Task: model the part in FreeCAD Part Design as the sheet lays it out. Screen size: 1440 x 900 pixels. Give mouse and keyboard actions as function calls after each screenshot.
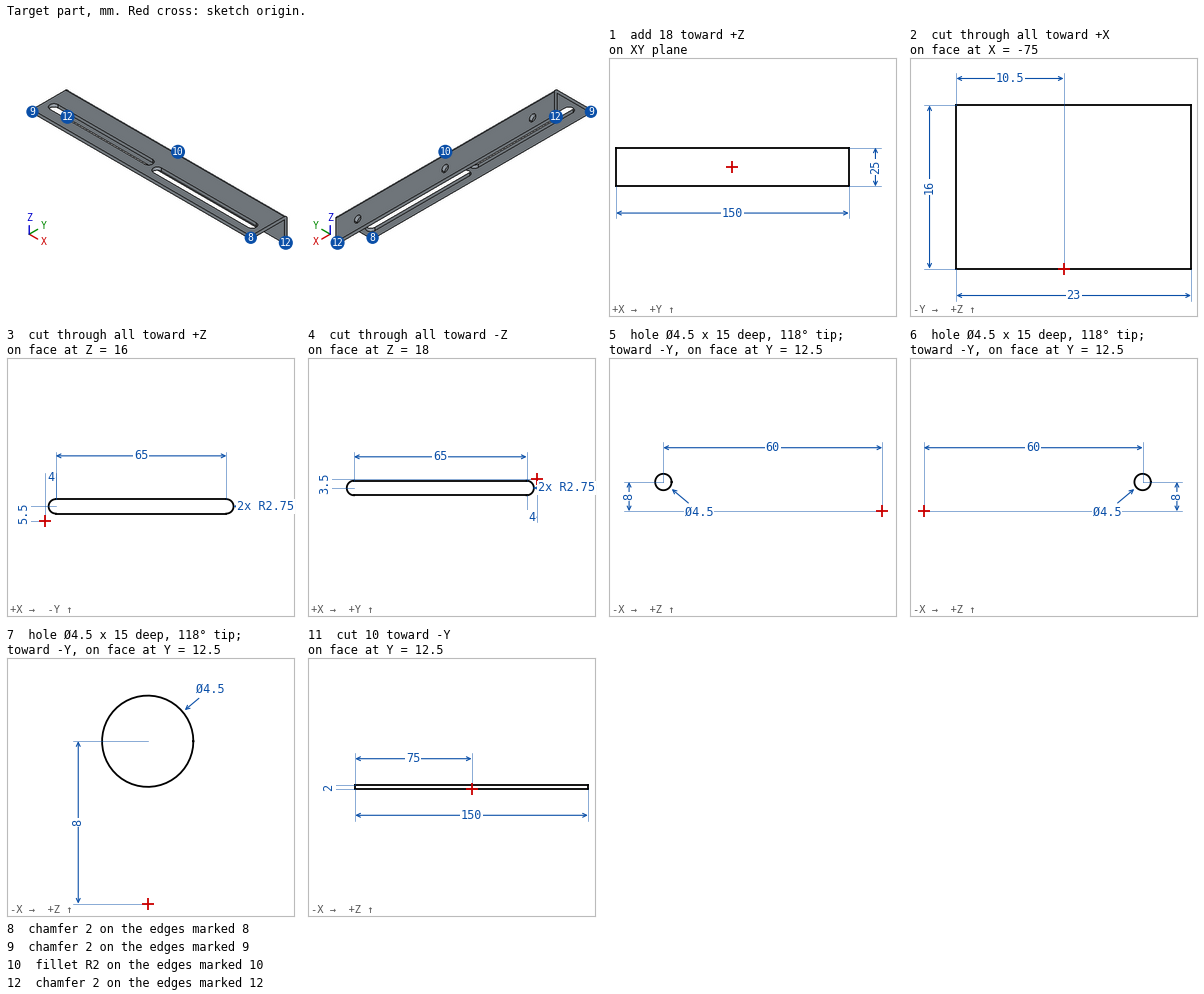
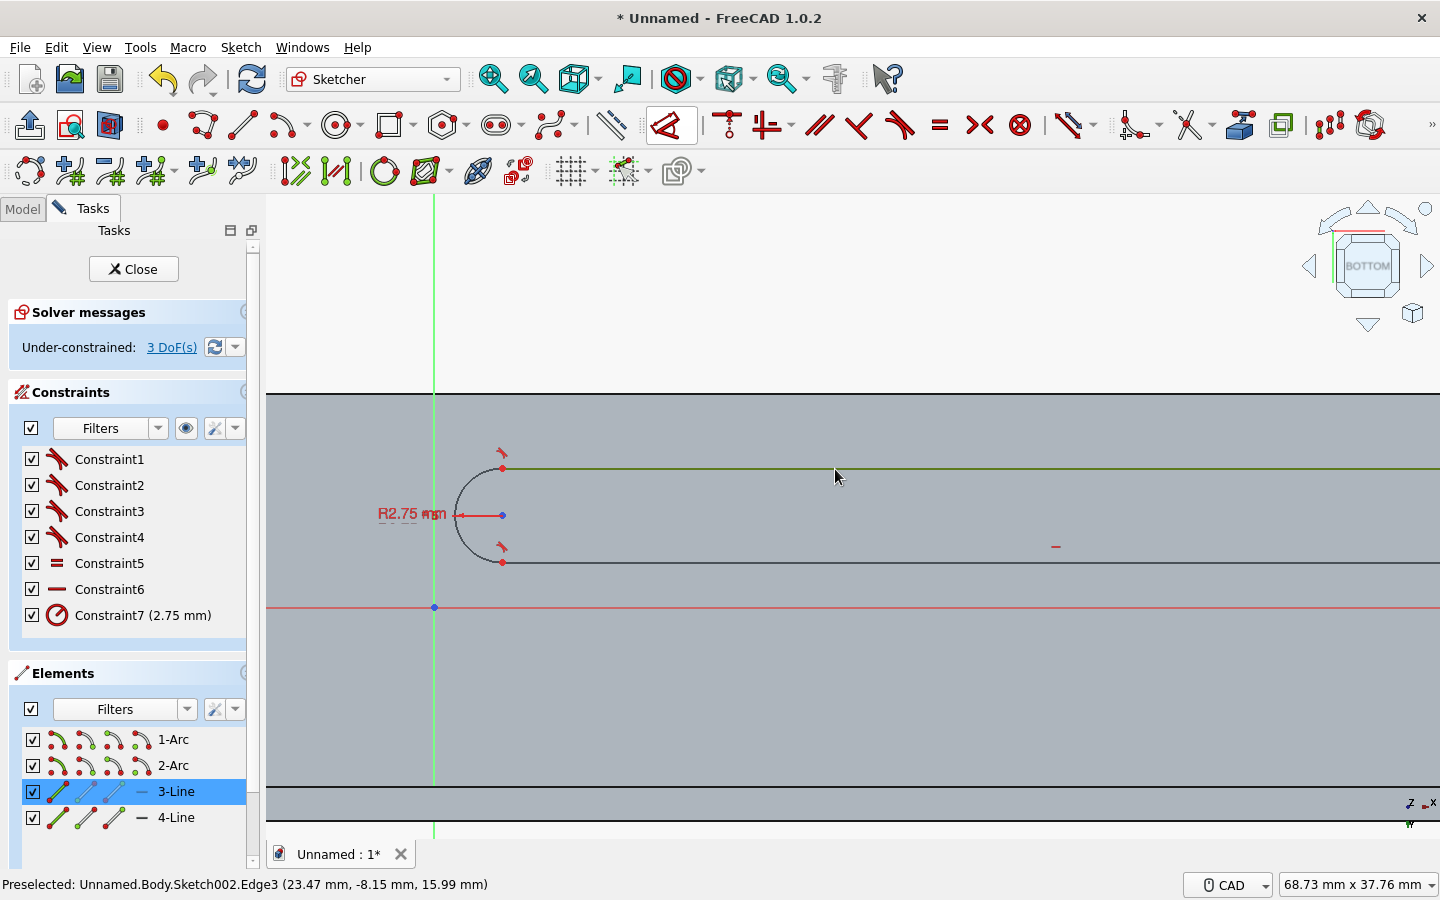
key(l)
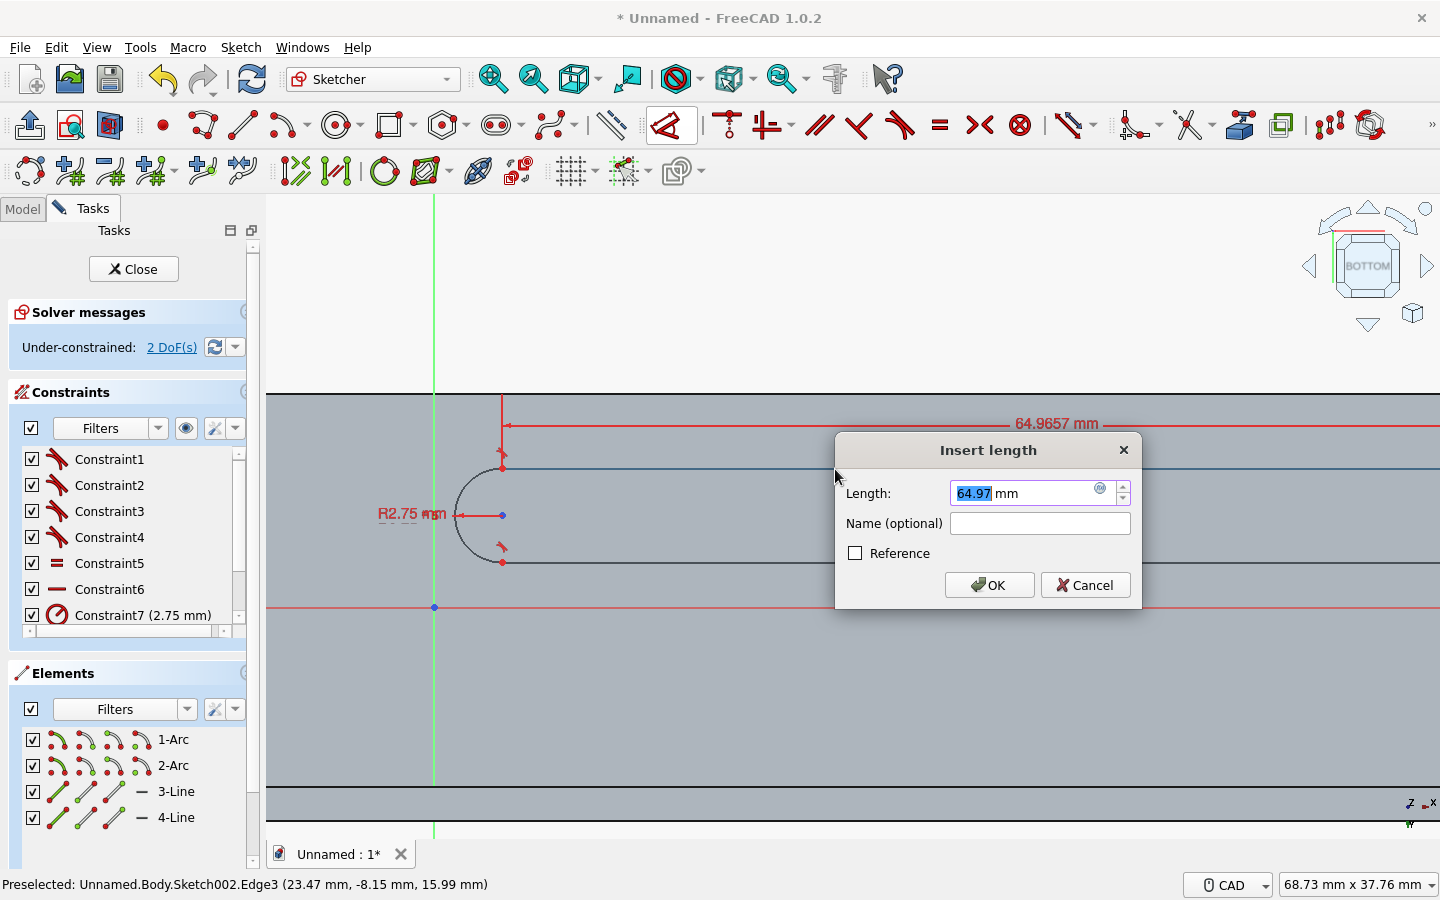
text(65)
key(Return)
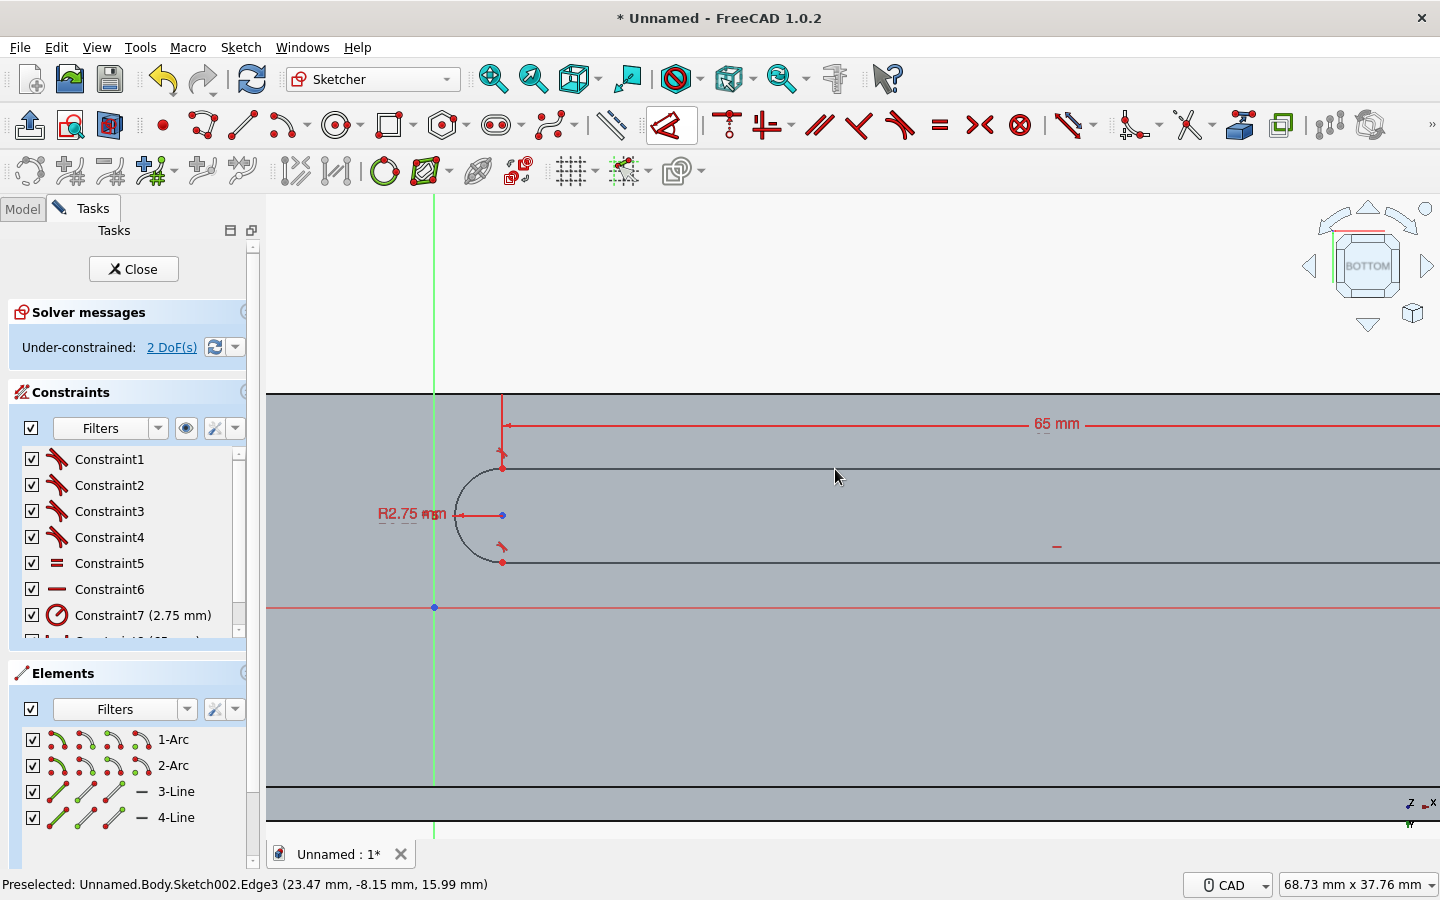
click(502, 469)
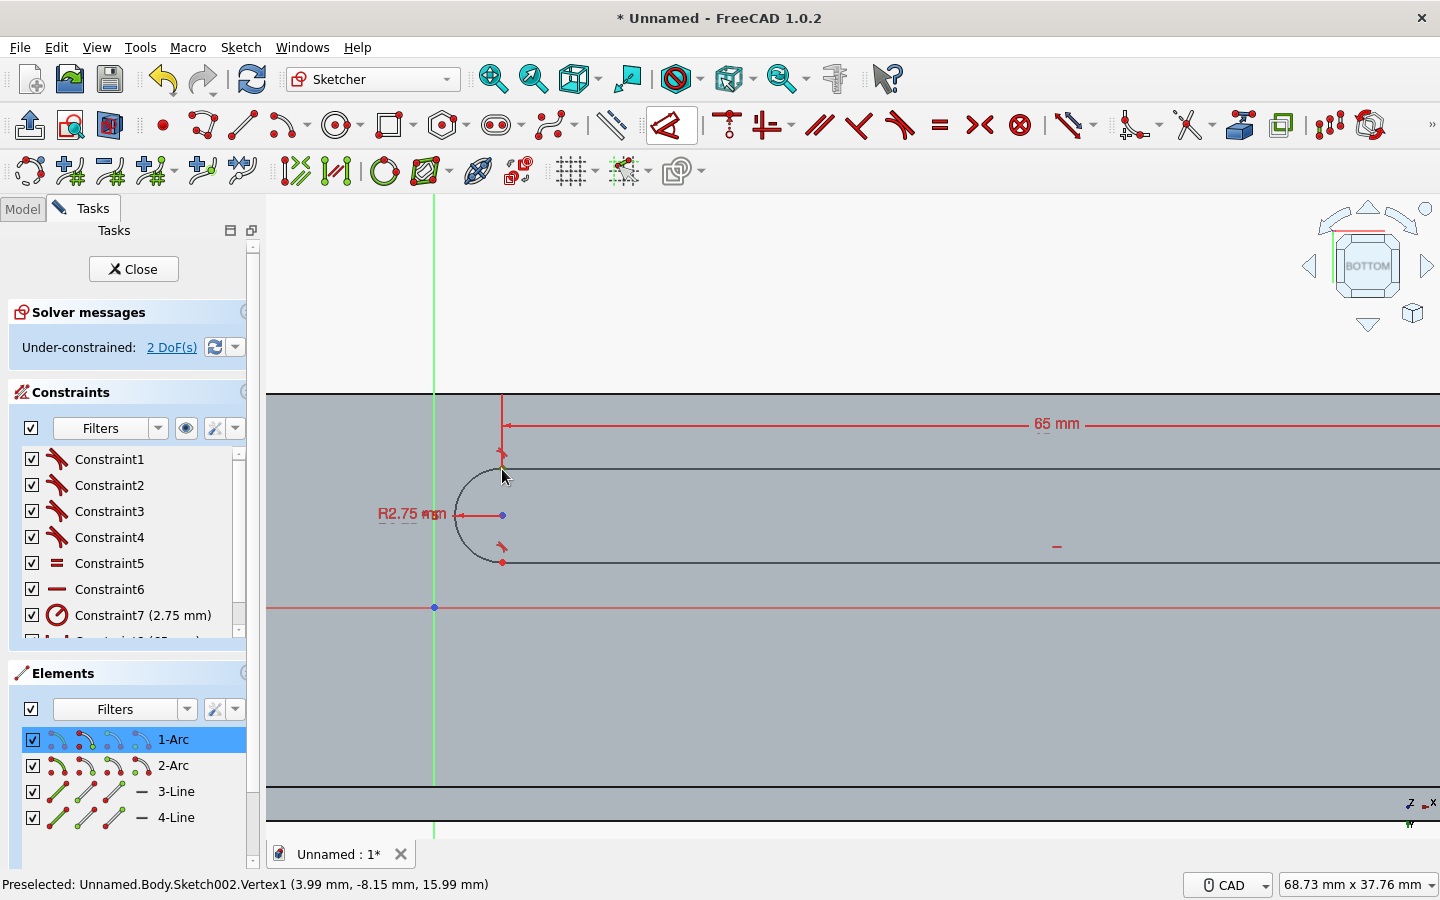
click(692, 126)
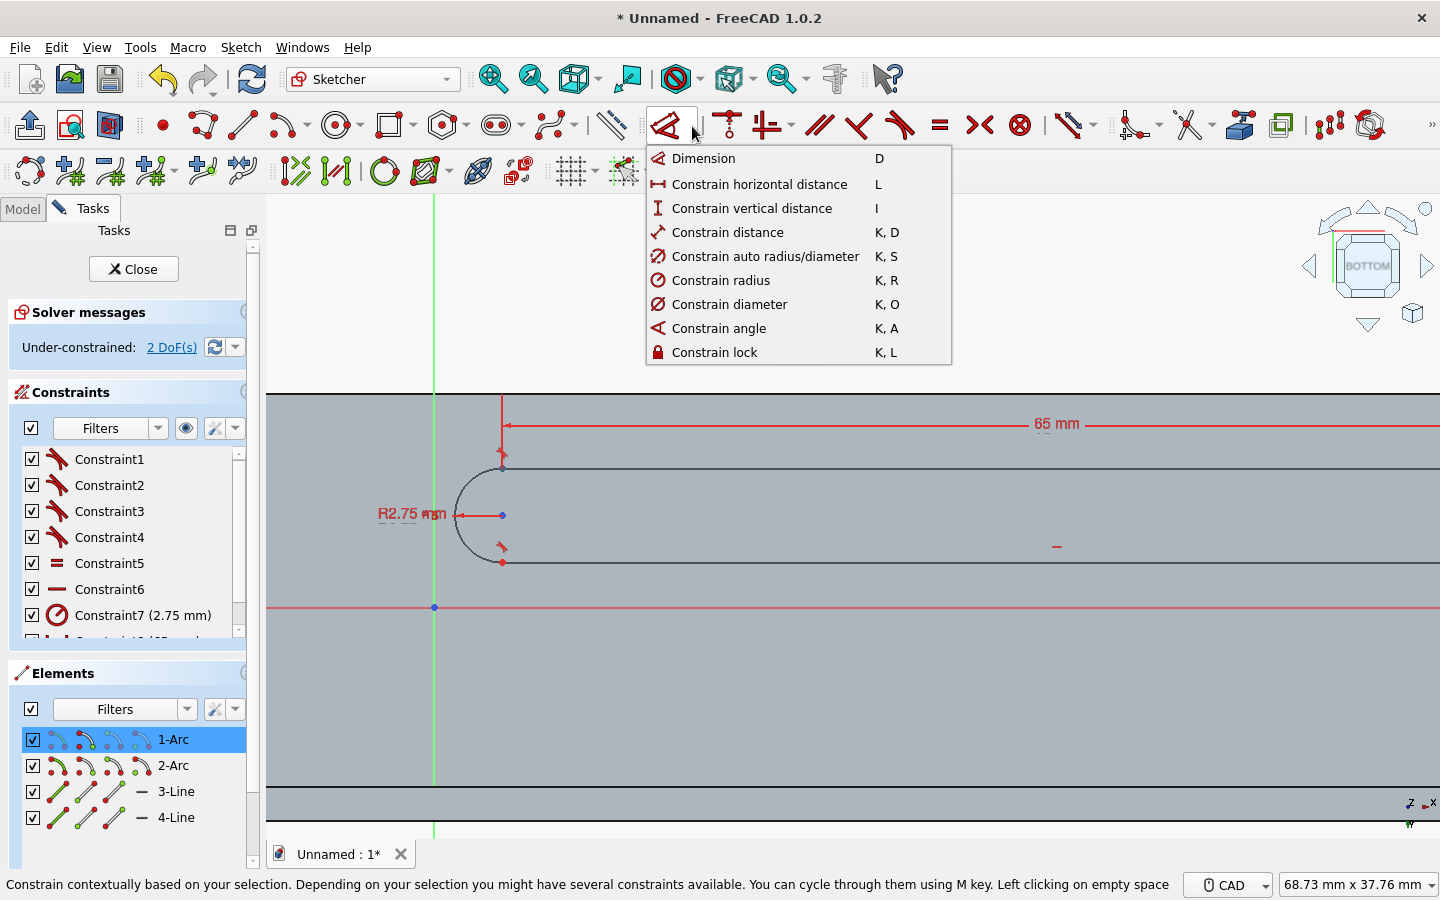
click(799, 184)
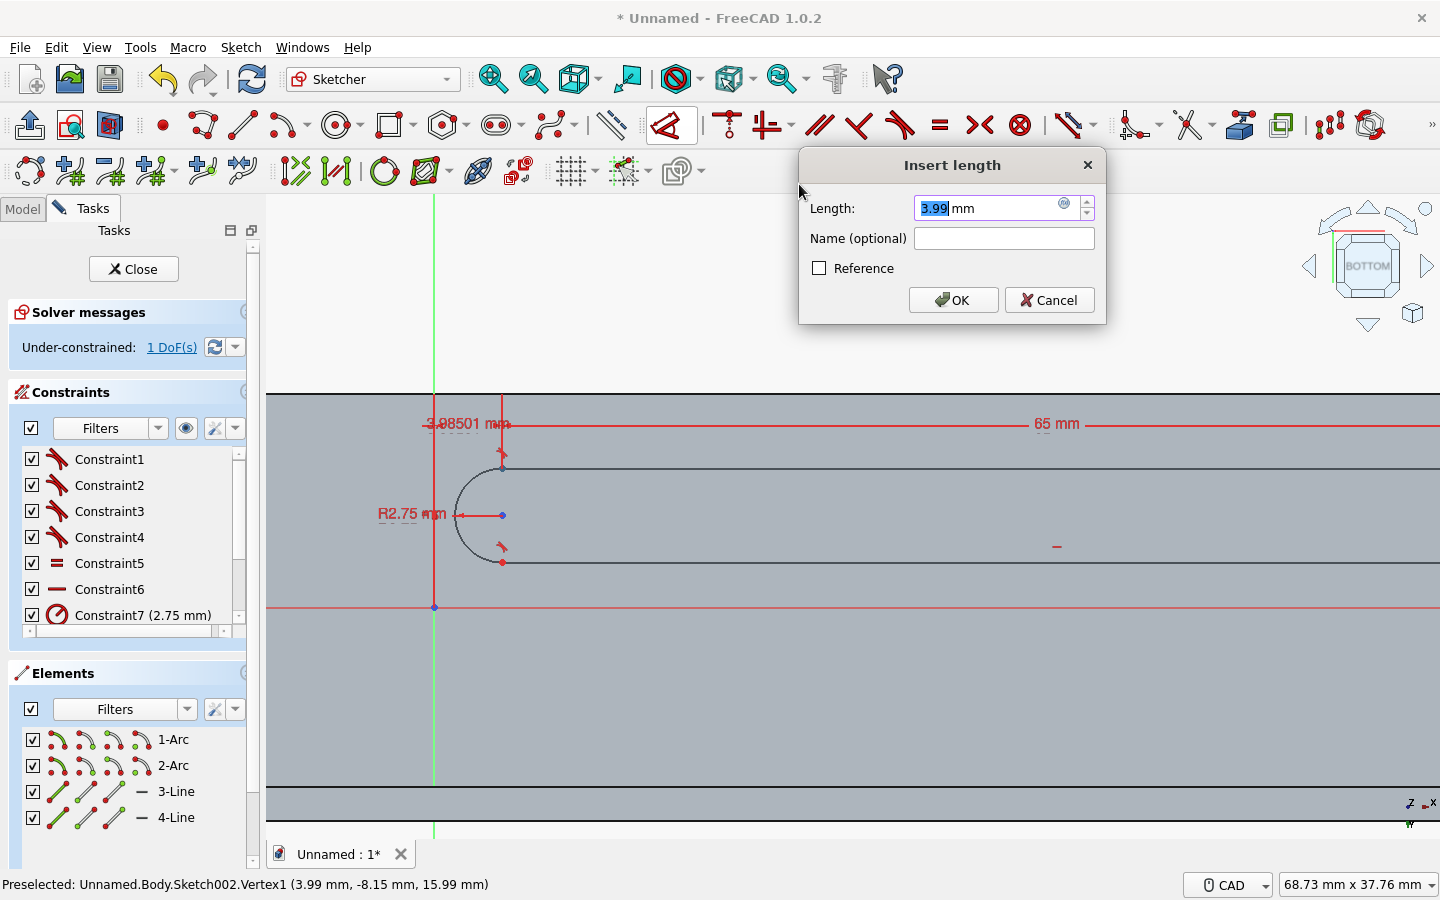
text(4)
key(Return)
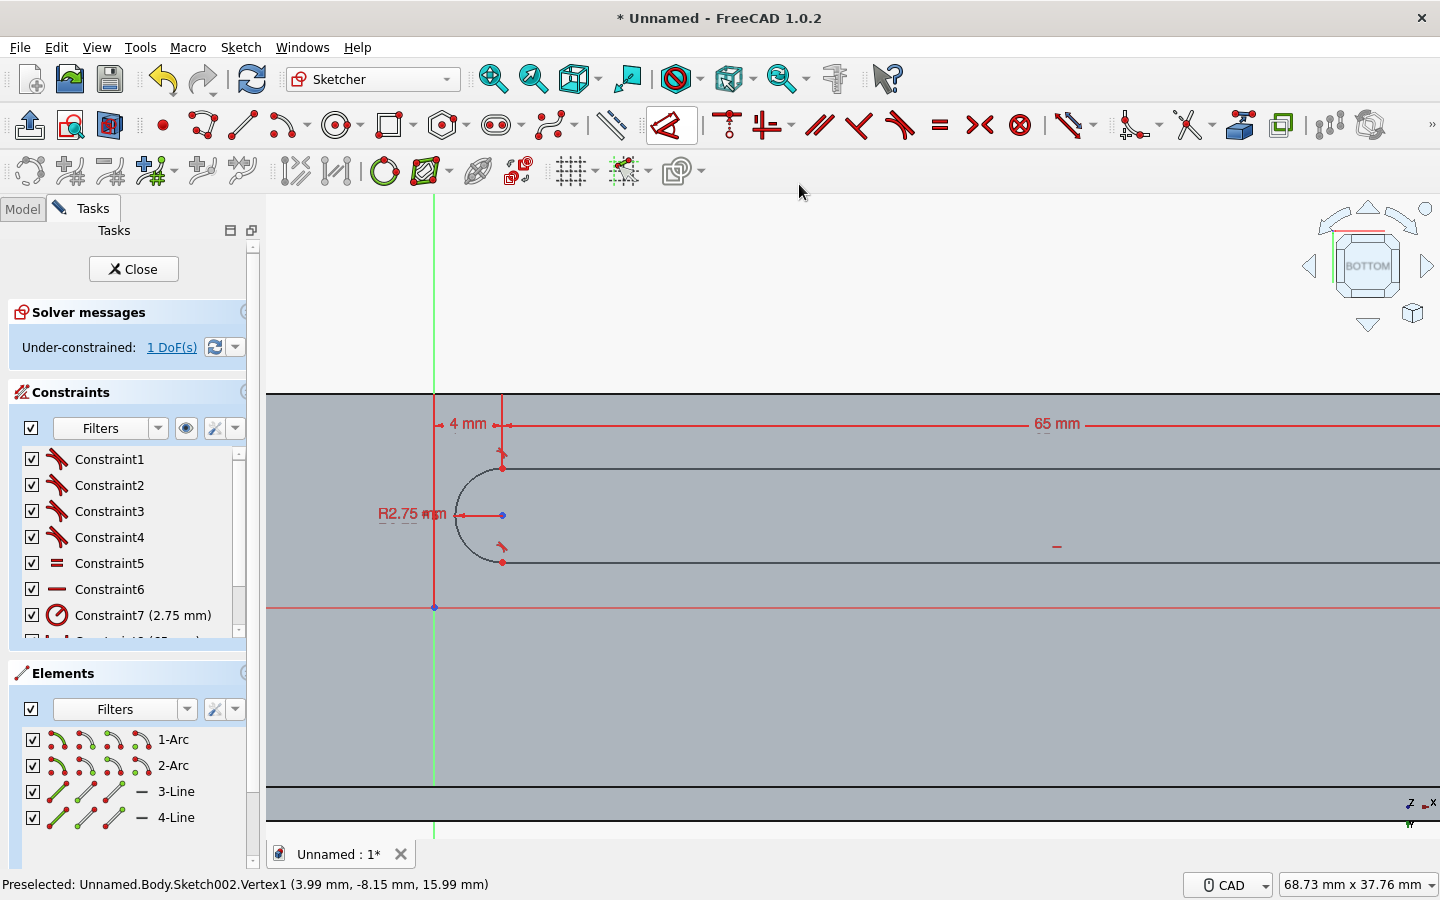
click(502, 516)